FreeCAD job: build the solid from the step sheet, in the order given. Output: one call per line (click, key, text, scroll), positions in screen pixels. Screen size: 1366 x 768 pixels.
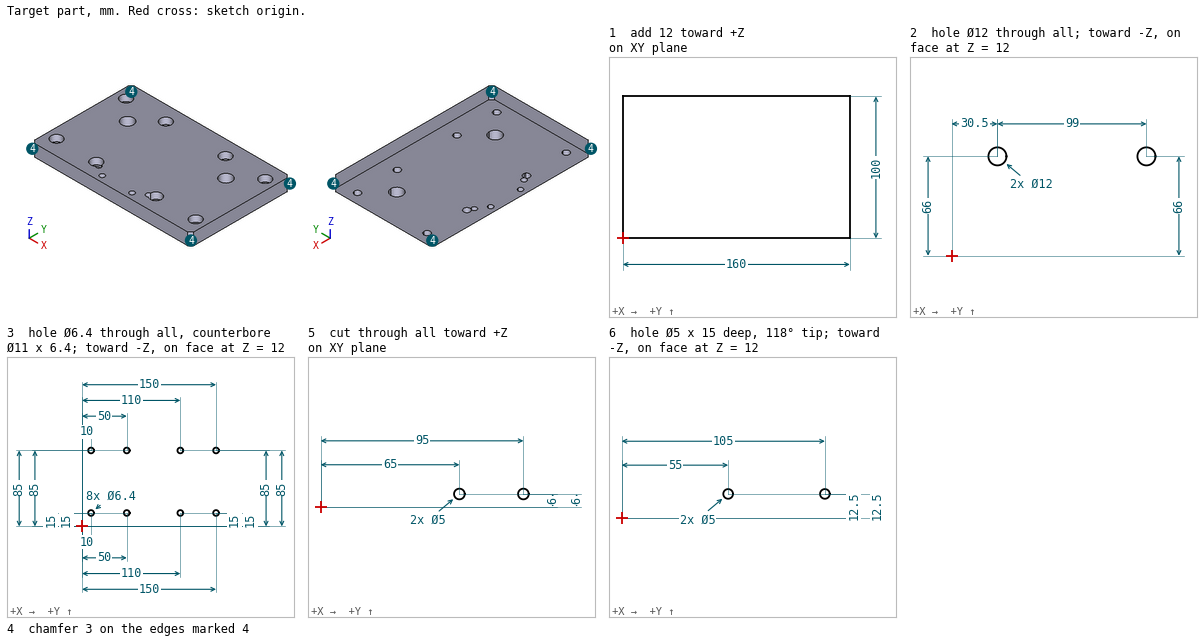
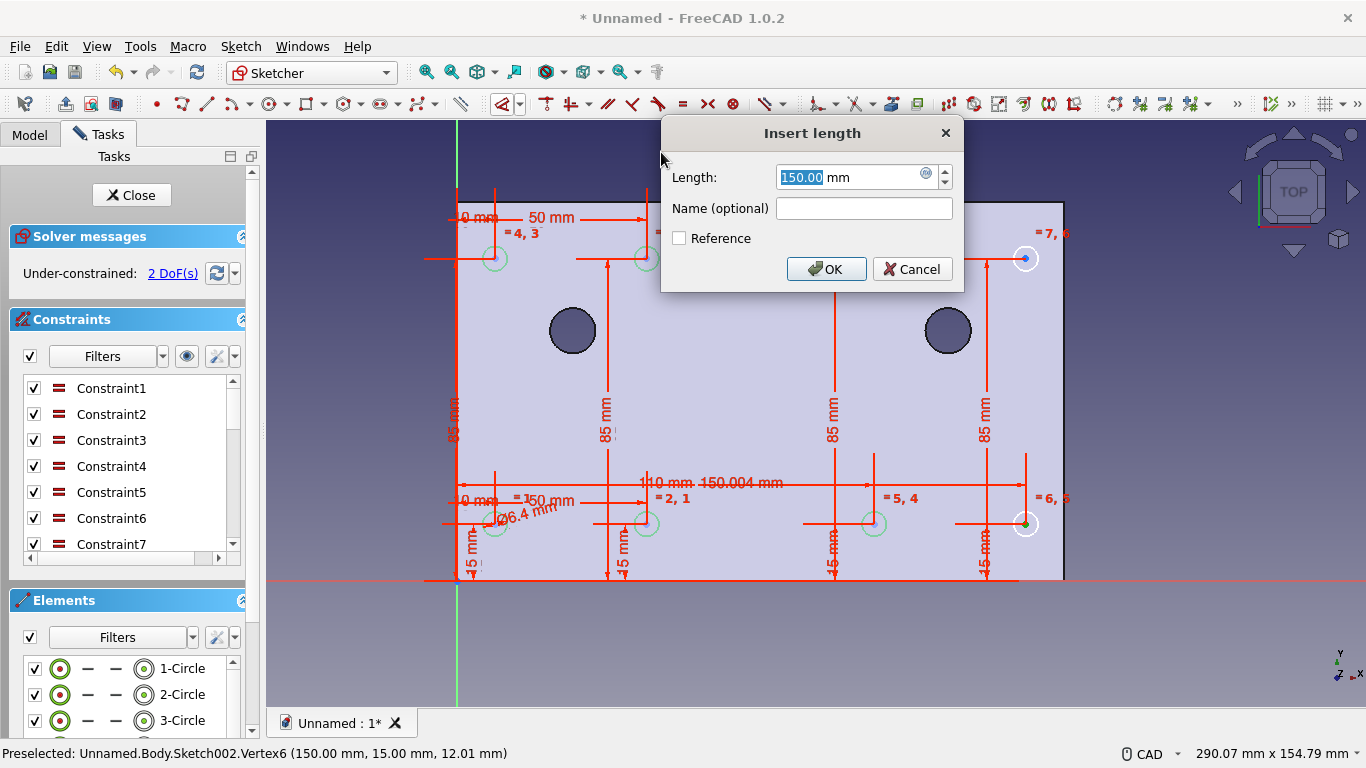
text(150)
key(Return)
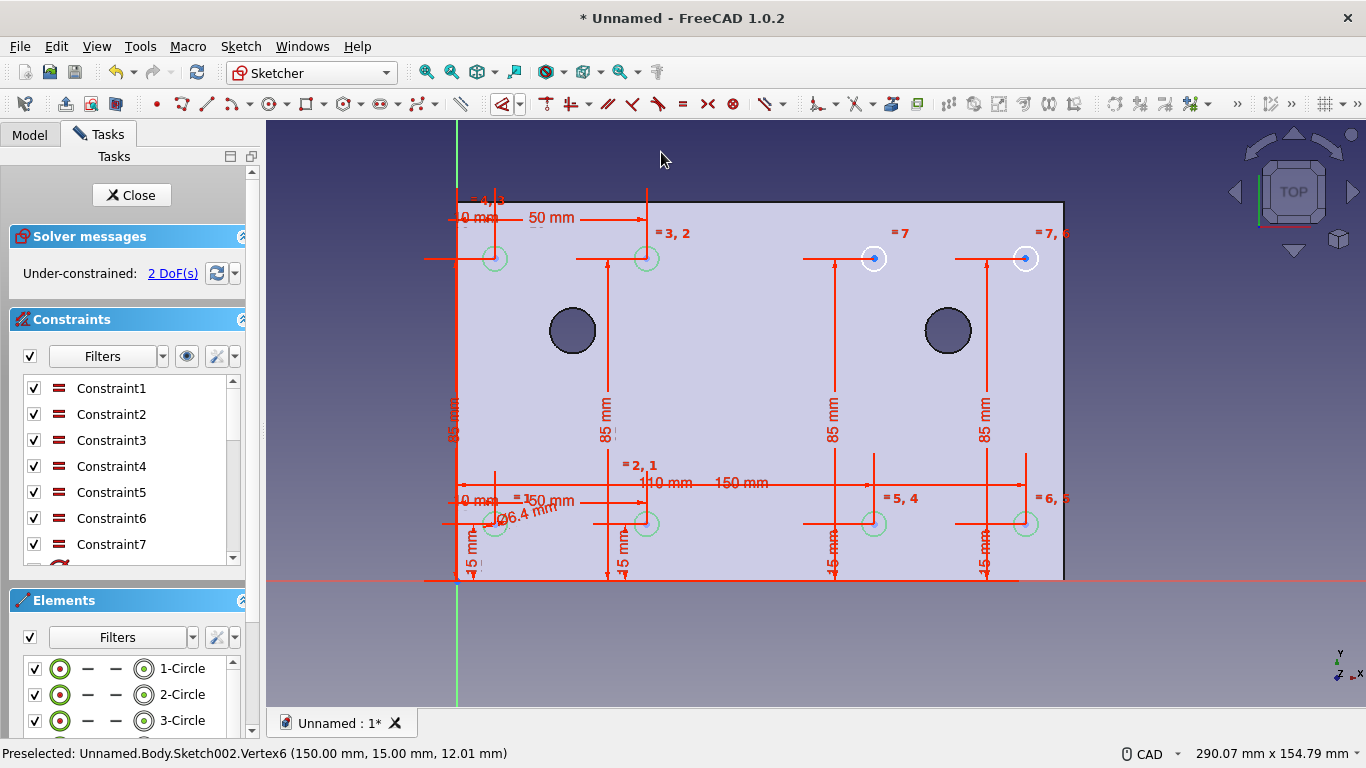
click(1026, 259)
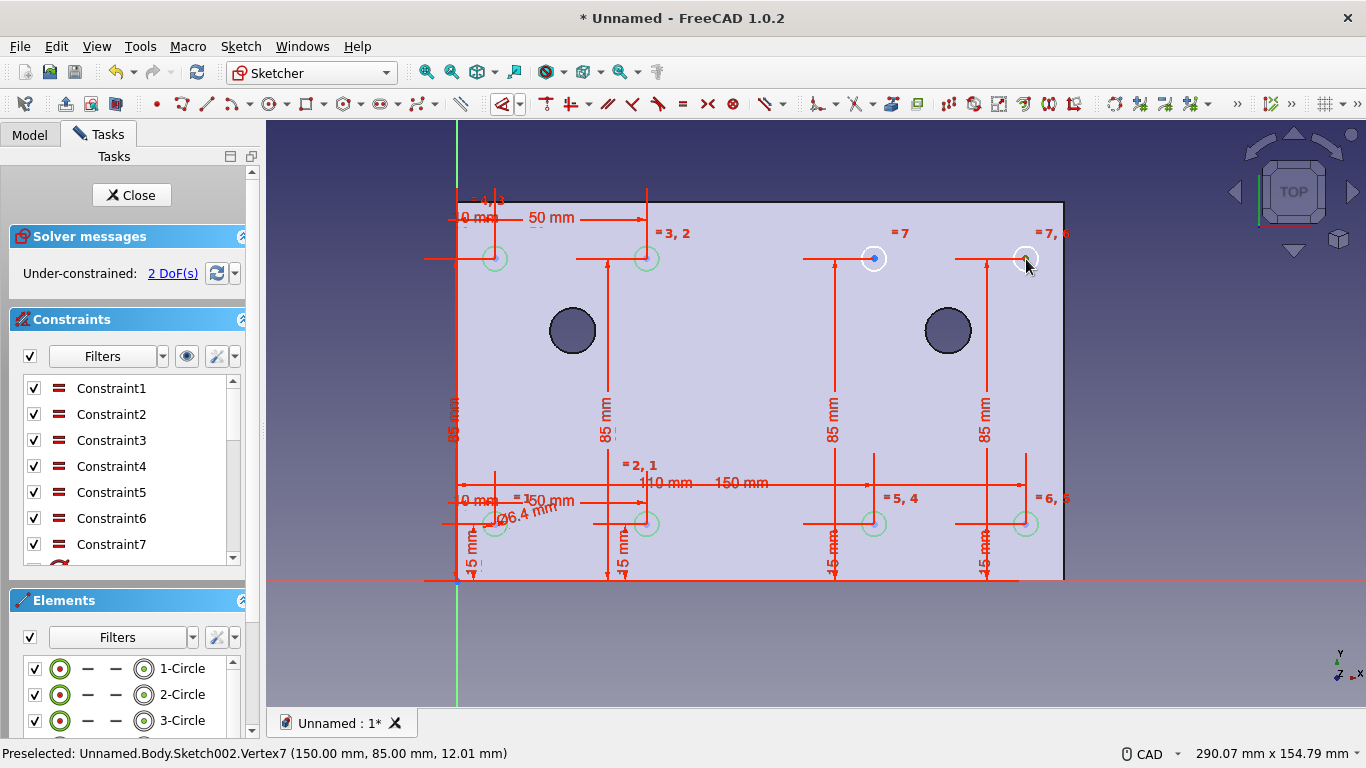
key(l)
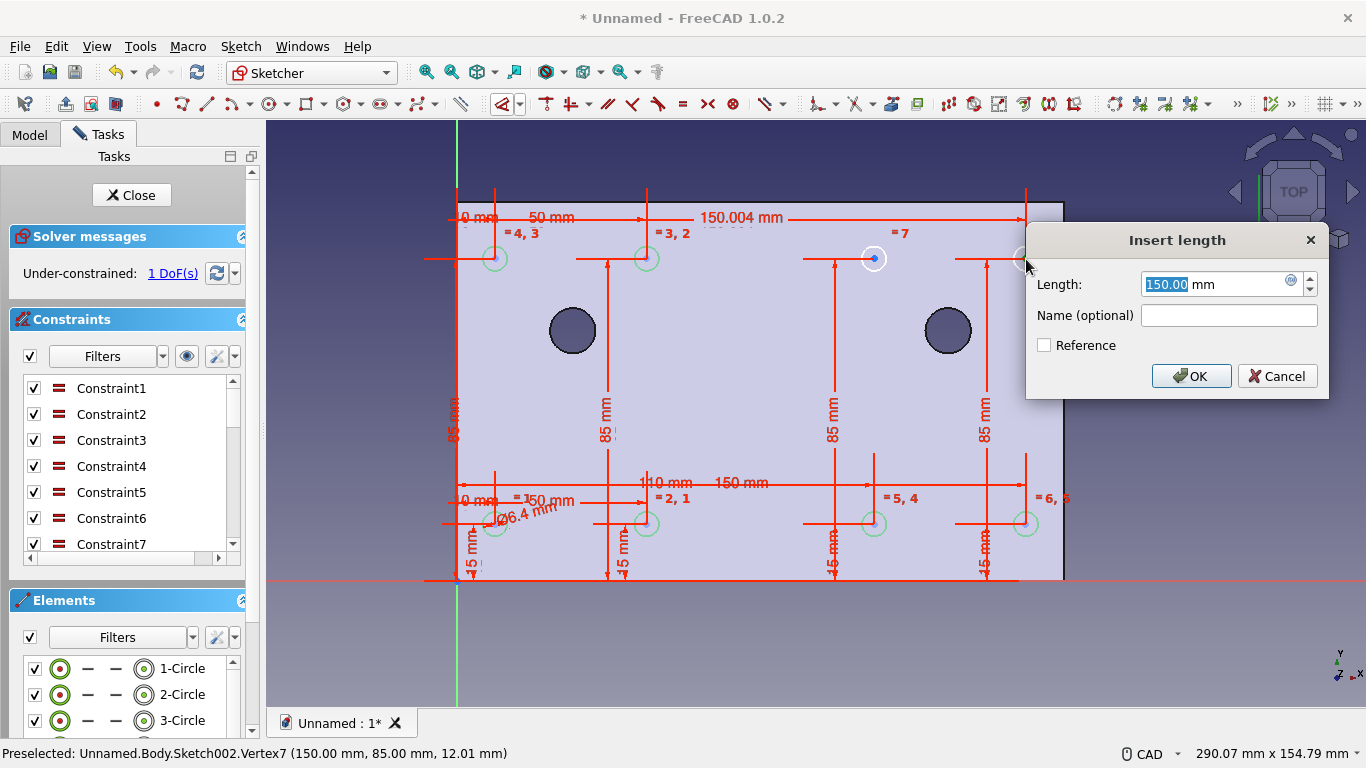
text(150)
key(Return)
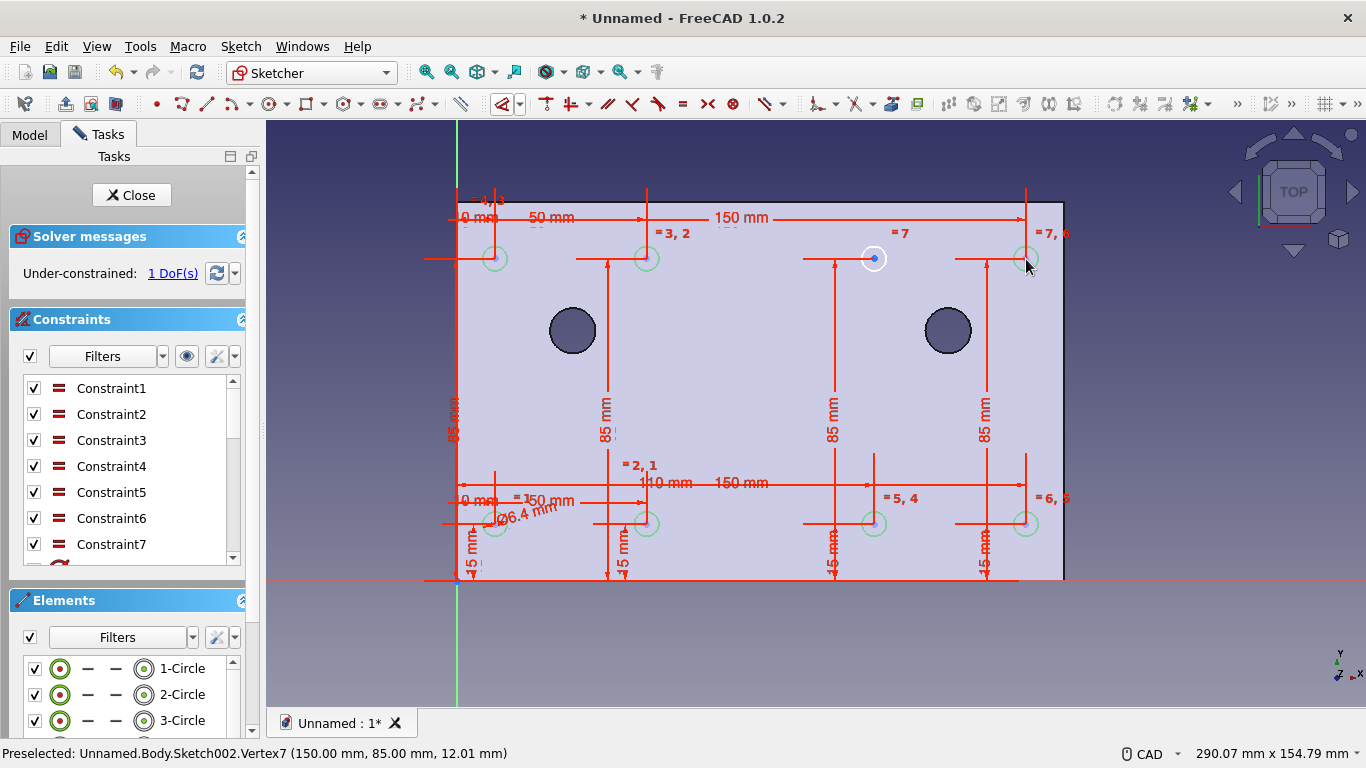
click(874, 259)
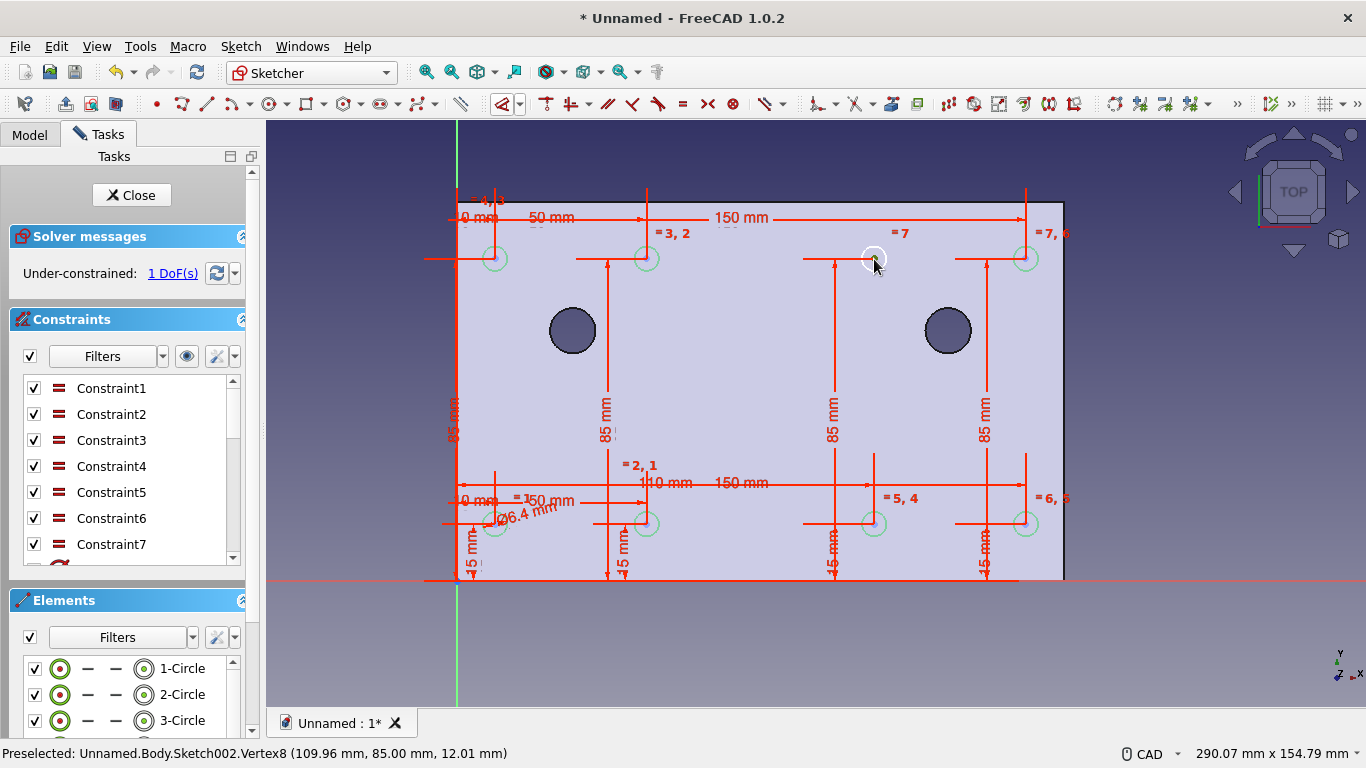
key(l)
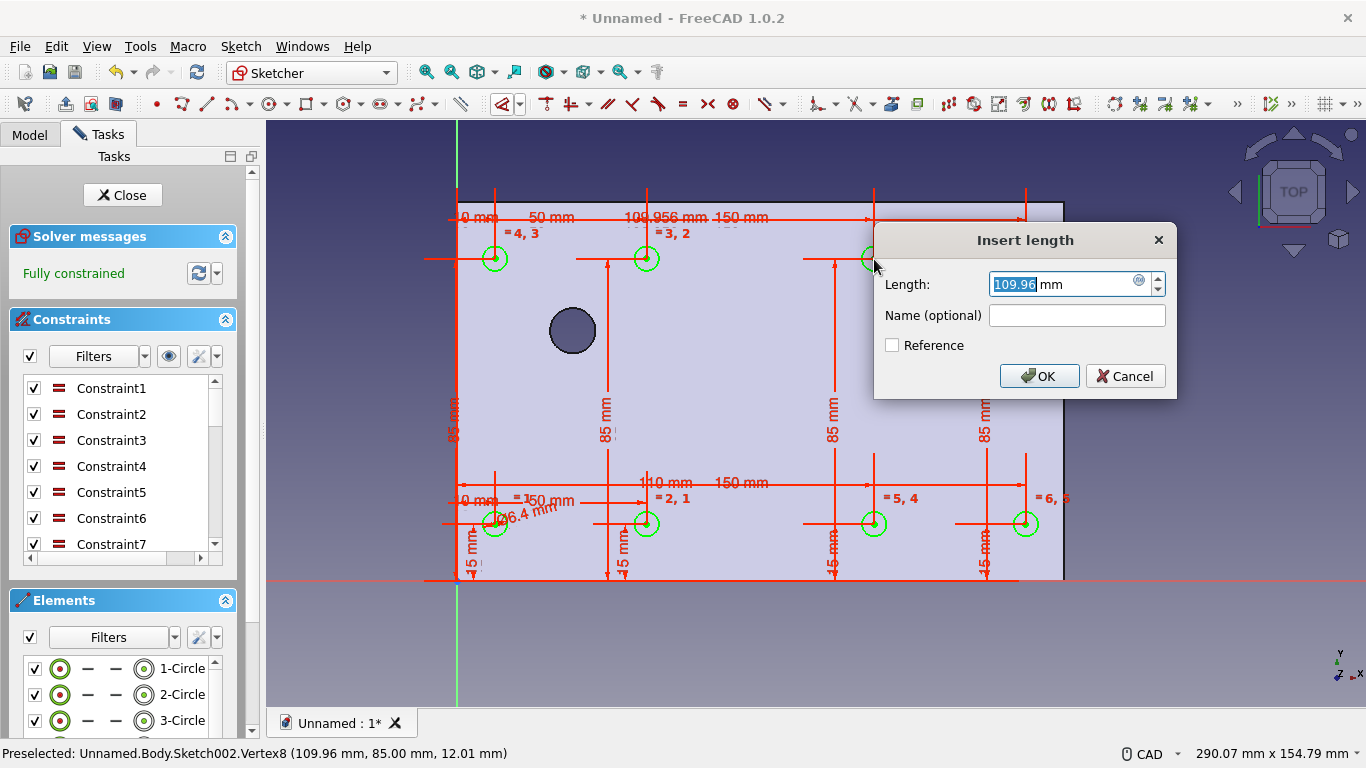
text(110)
key(Return)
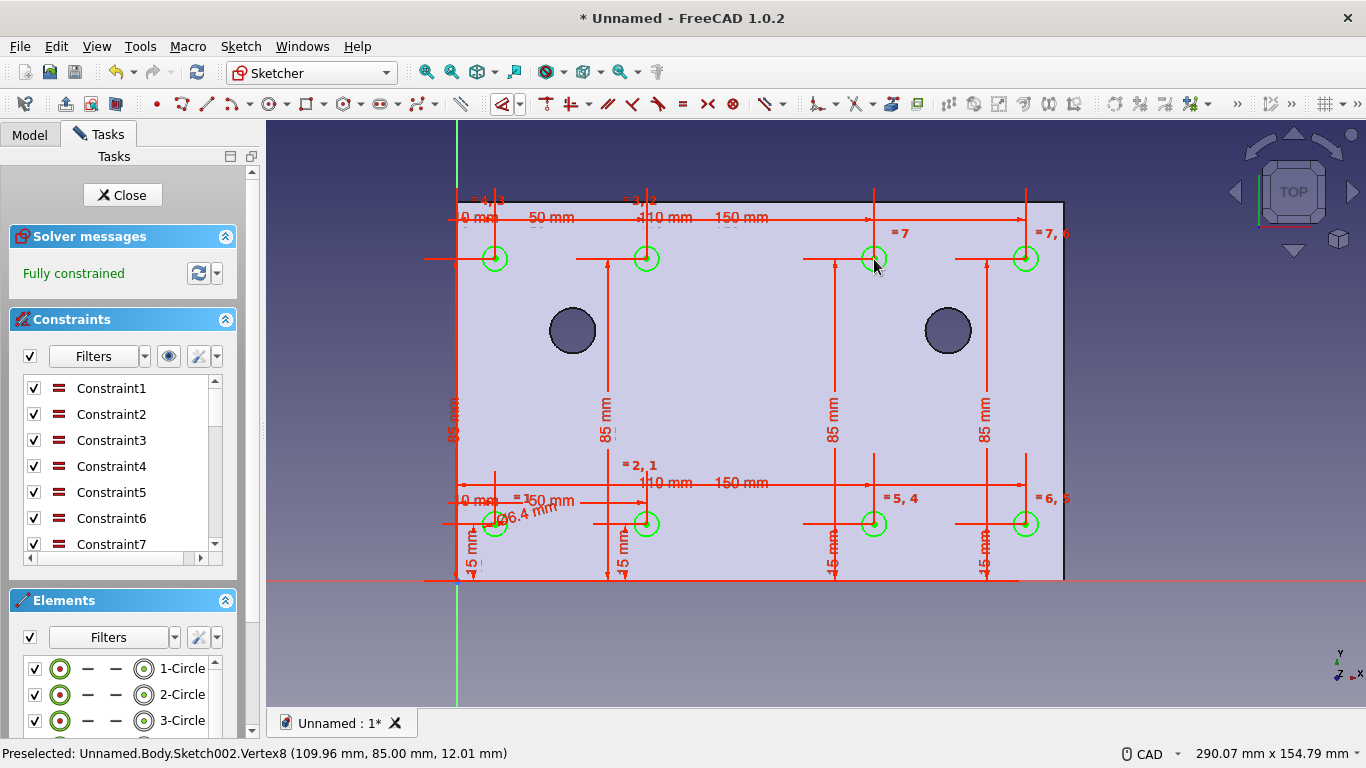
click(123, 195)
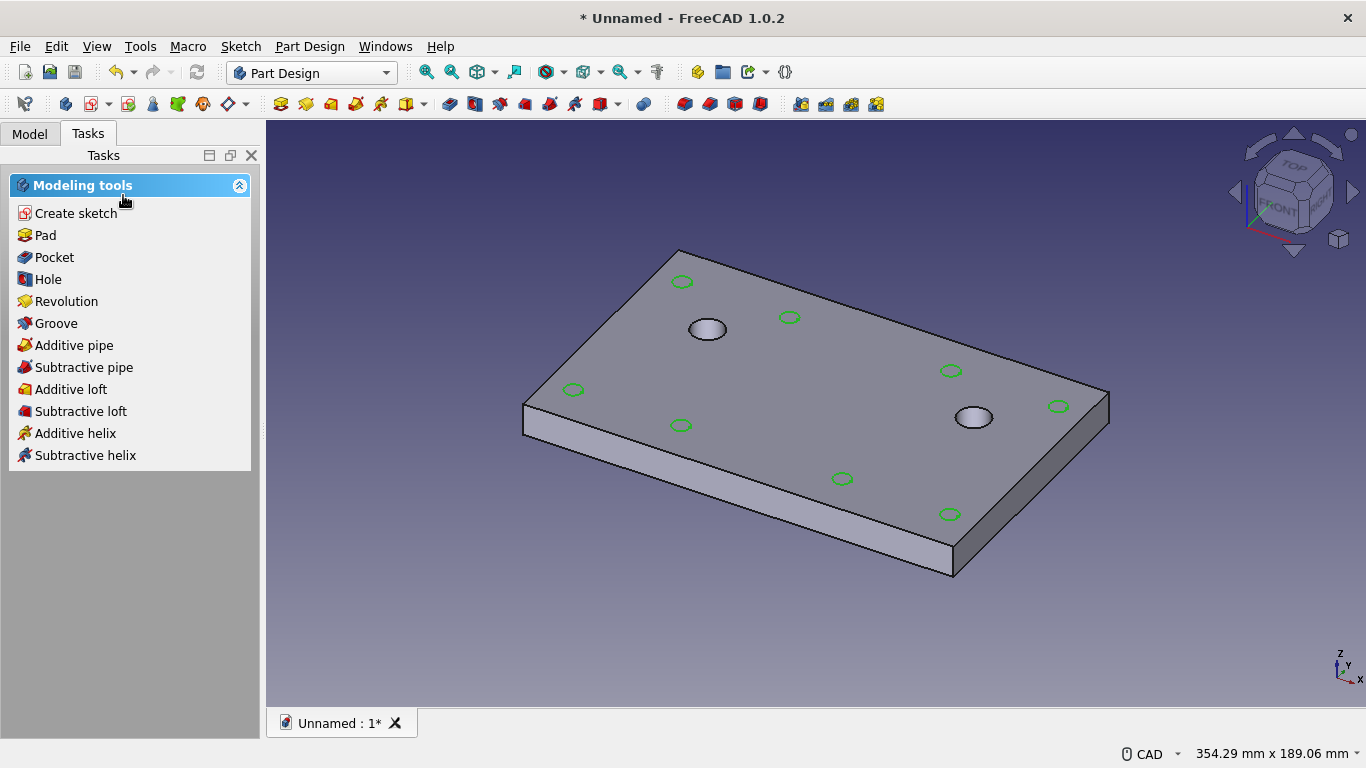
click(475, 104)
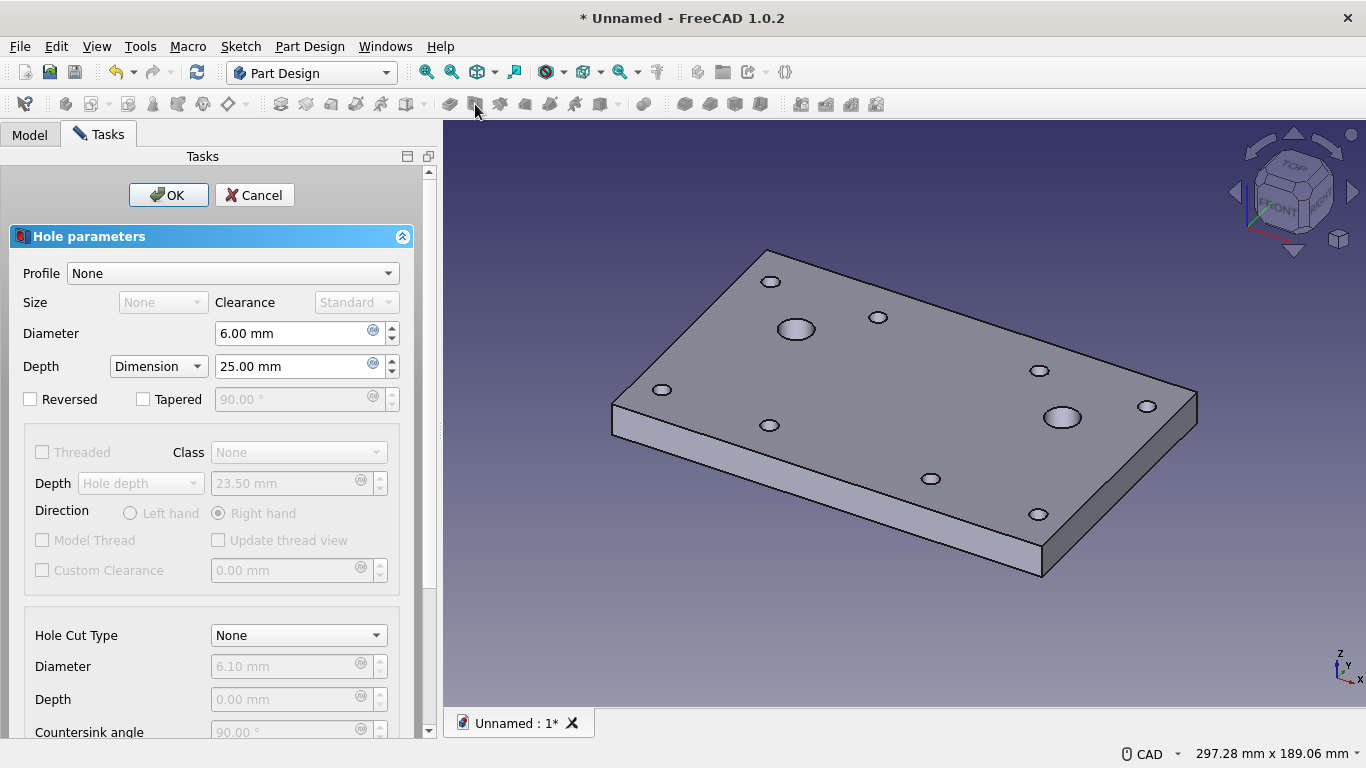
triple_click(300, 334)